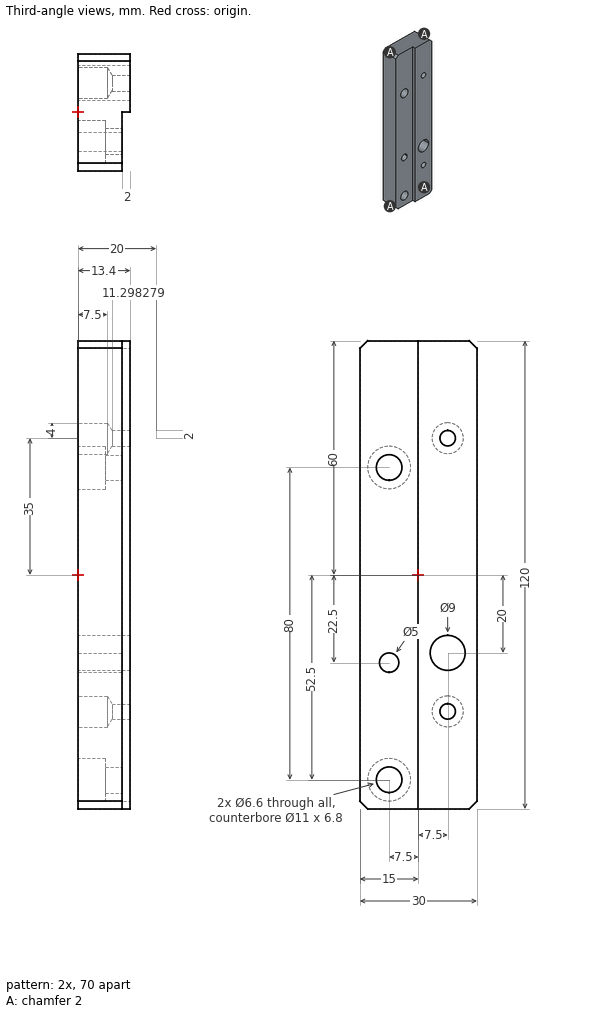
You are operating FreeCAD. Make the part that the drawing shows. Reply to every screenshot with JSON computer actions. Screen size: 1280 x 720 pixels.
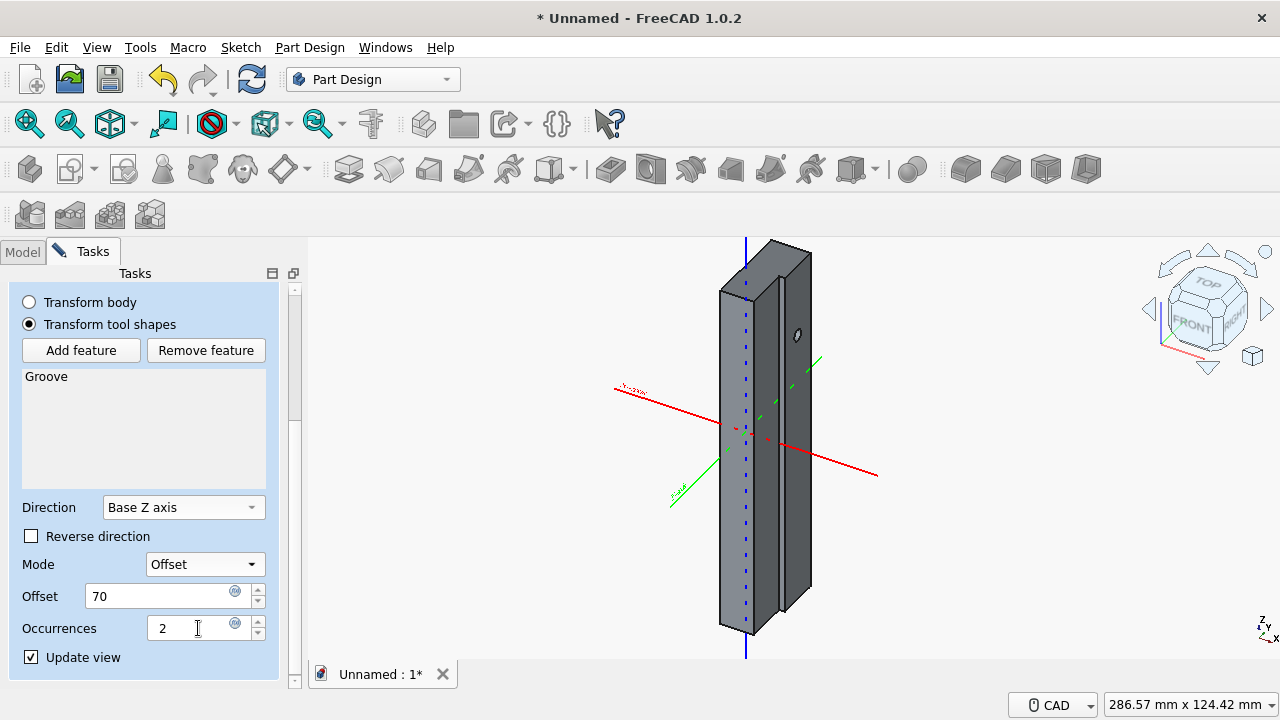
{"action": "left_click", "coordinate": [30, 536]}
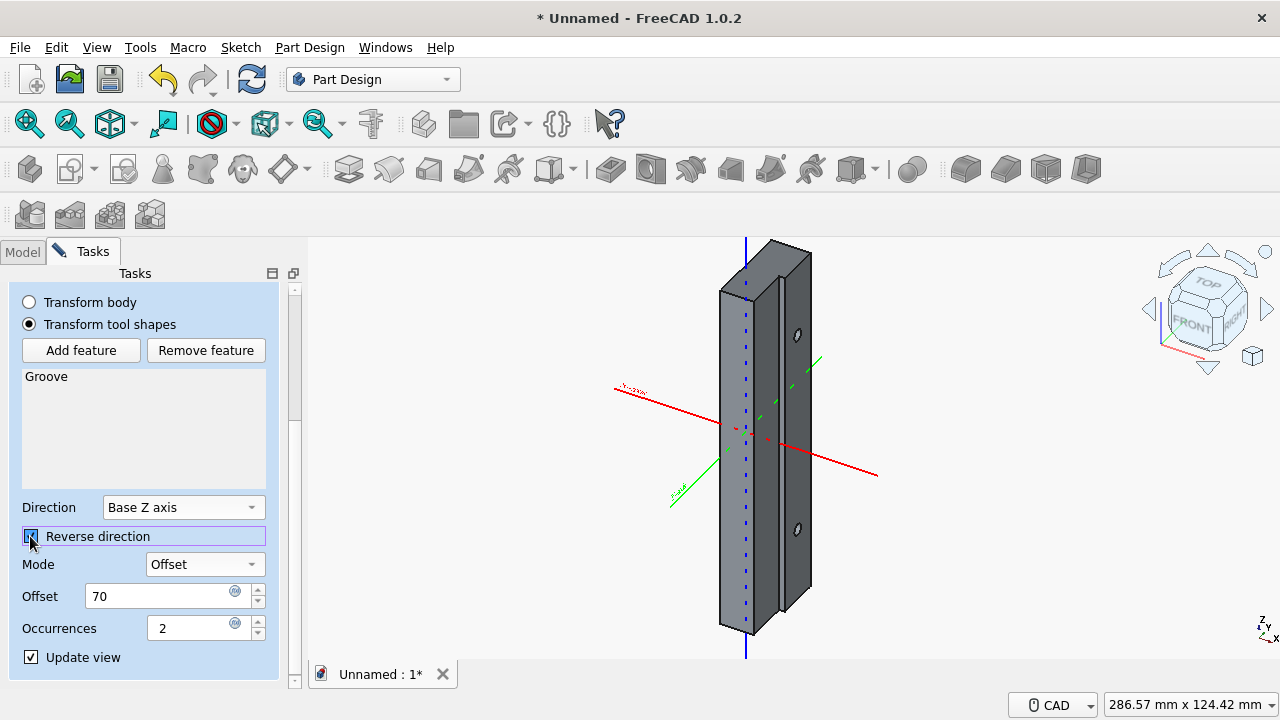
{"action": "scroll", "coordinate": [295, 486], "scroll_direction": "up", "scroll_amount": 5}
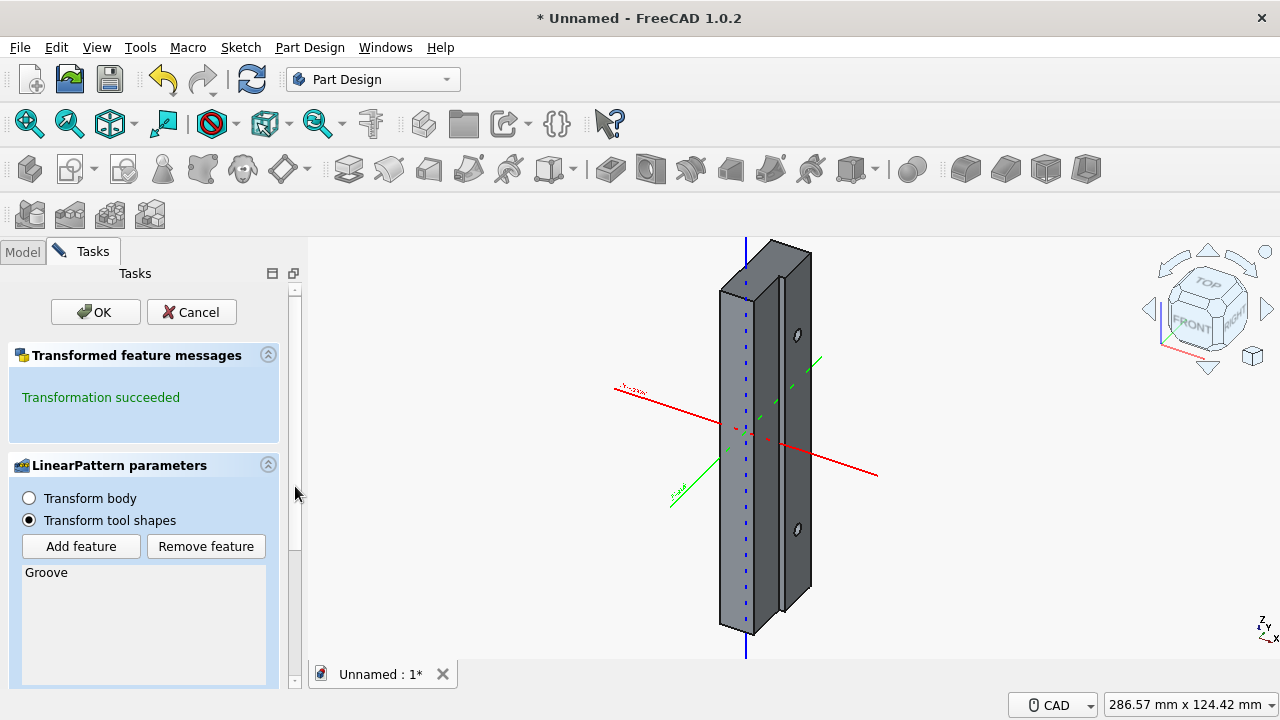
{"action": "left_click", "coordinate": [96, 312]}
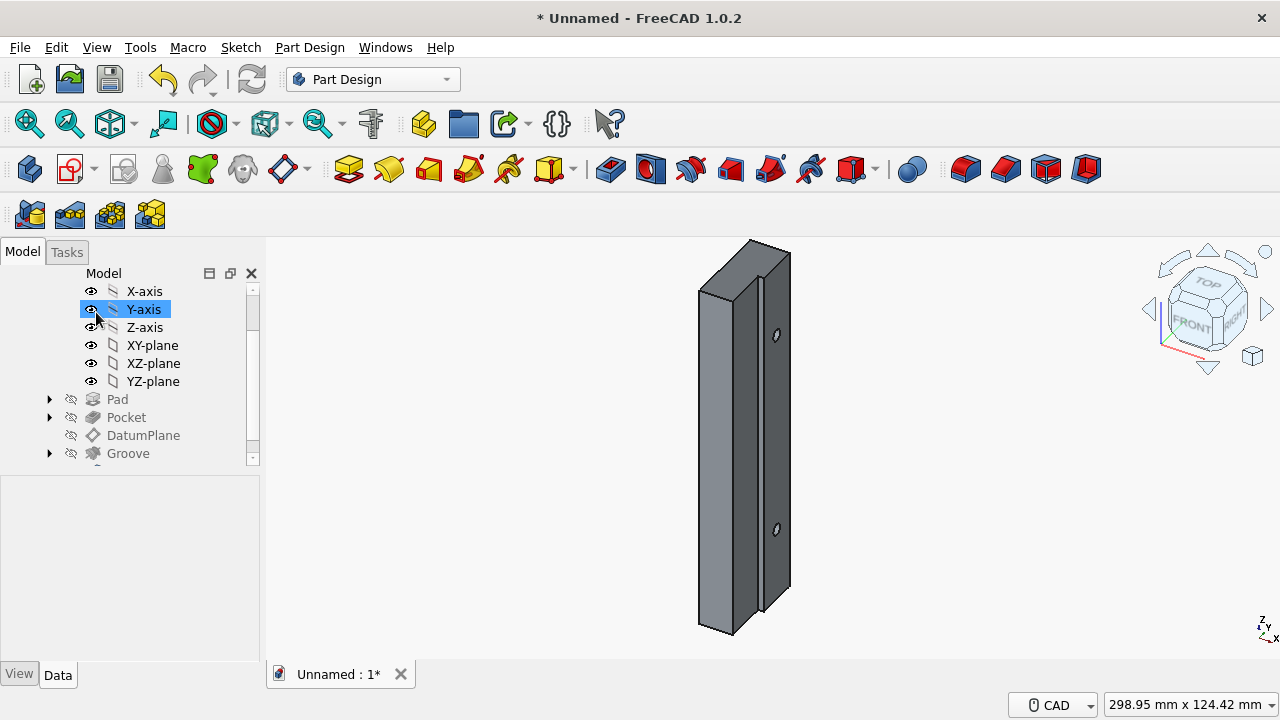
{"action": "left_click", "coordinate": [777, 289]}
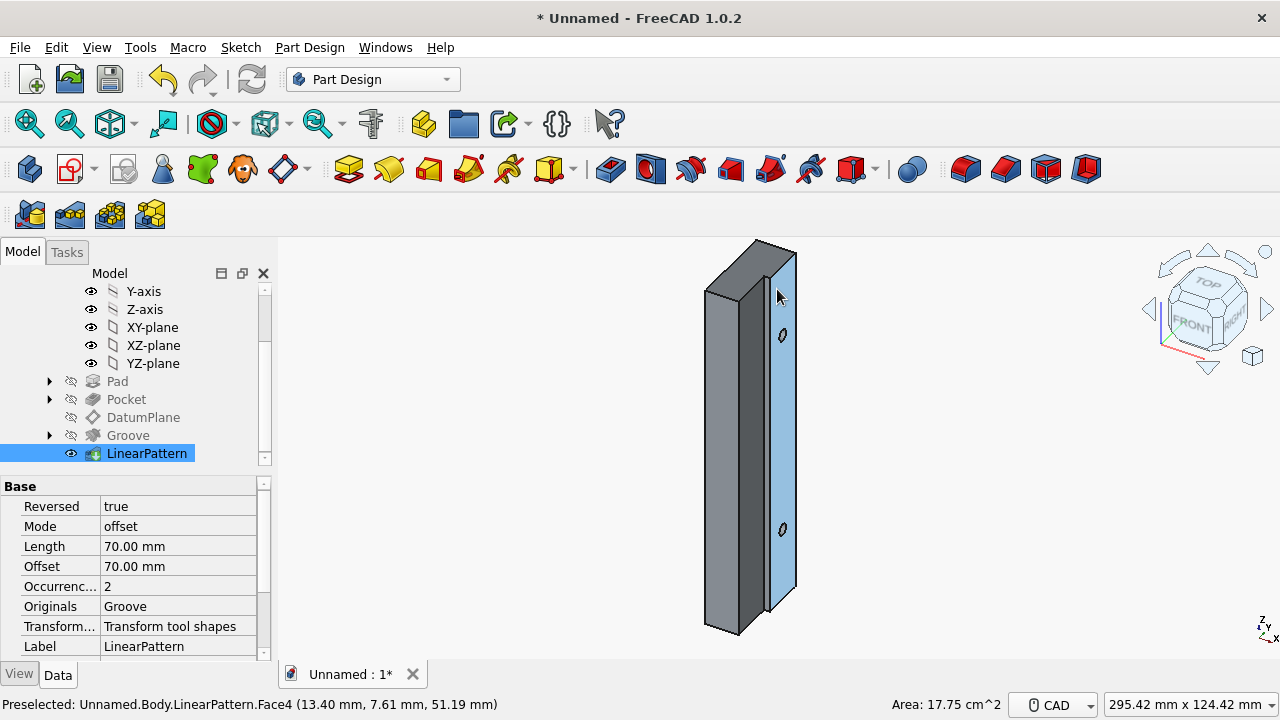
{"action": "left_click", "coordinate": [70, 170]}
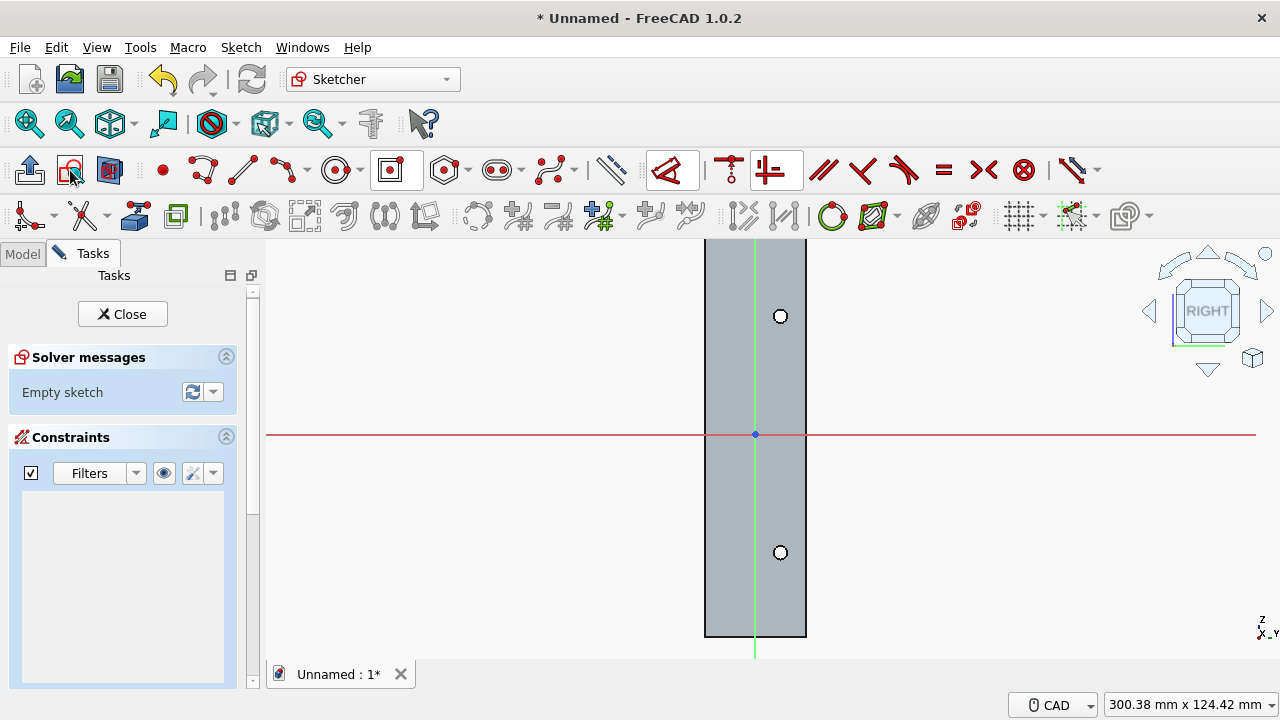
{"action": "scroll", "coordinate": [790, 509], "scroll_direction": "up", "scroll_amount": 11}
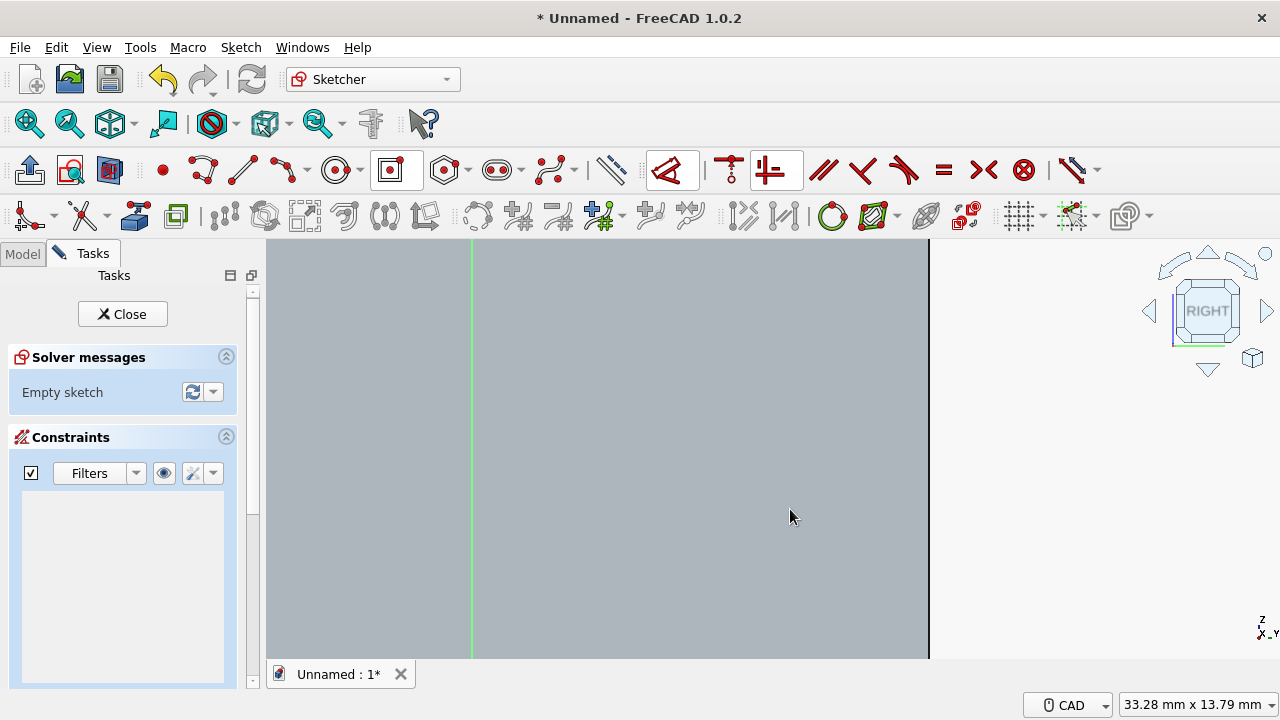
{"action": "left_click", "coordinate": [336, 170]}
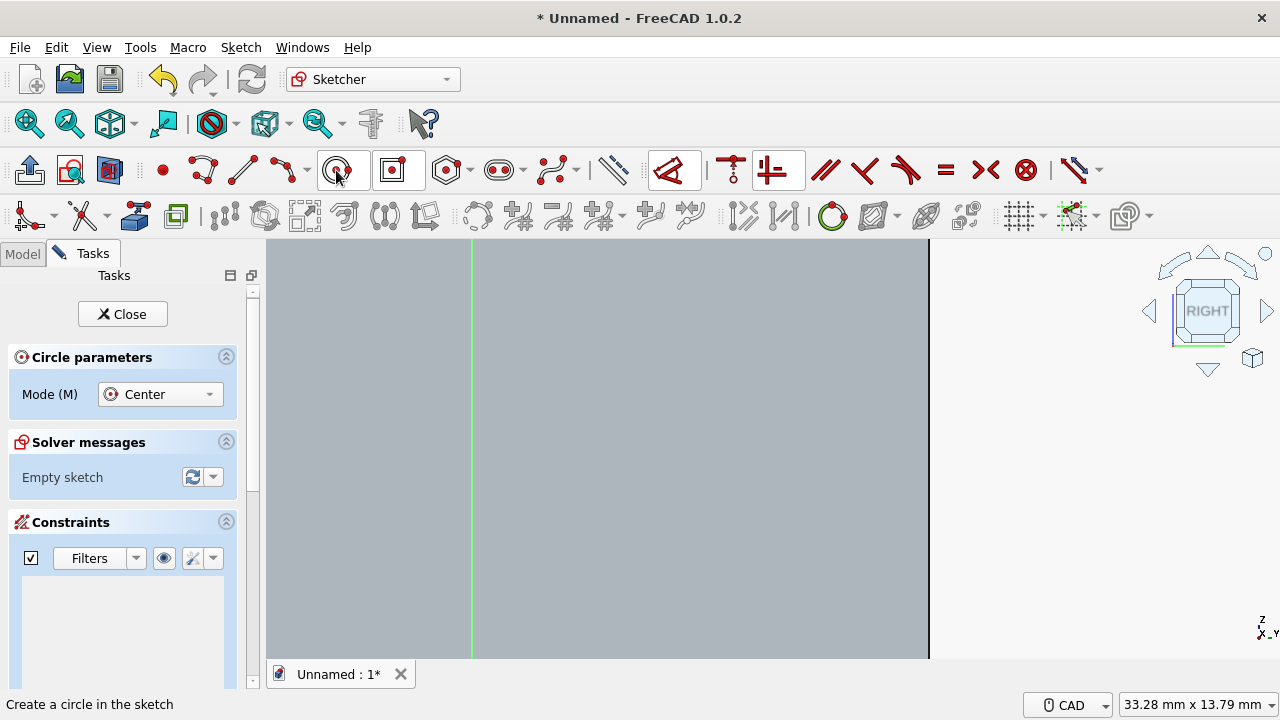
{"action": "left_click", "coordinate": [700, 442]}
{"action": "left_click", "coordinate": [797, 345]}
{"action": "key", "text": "Escape"}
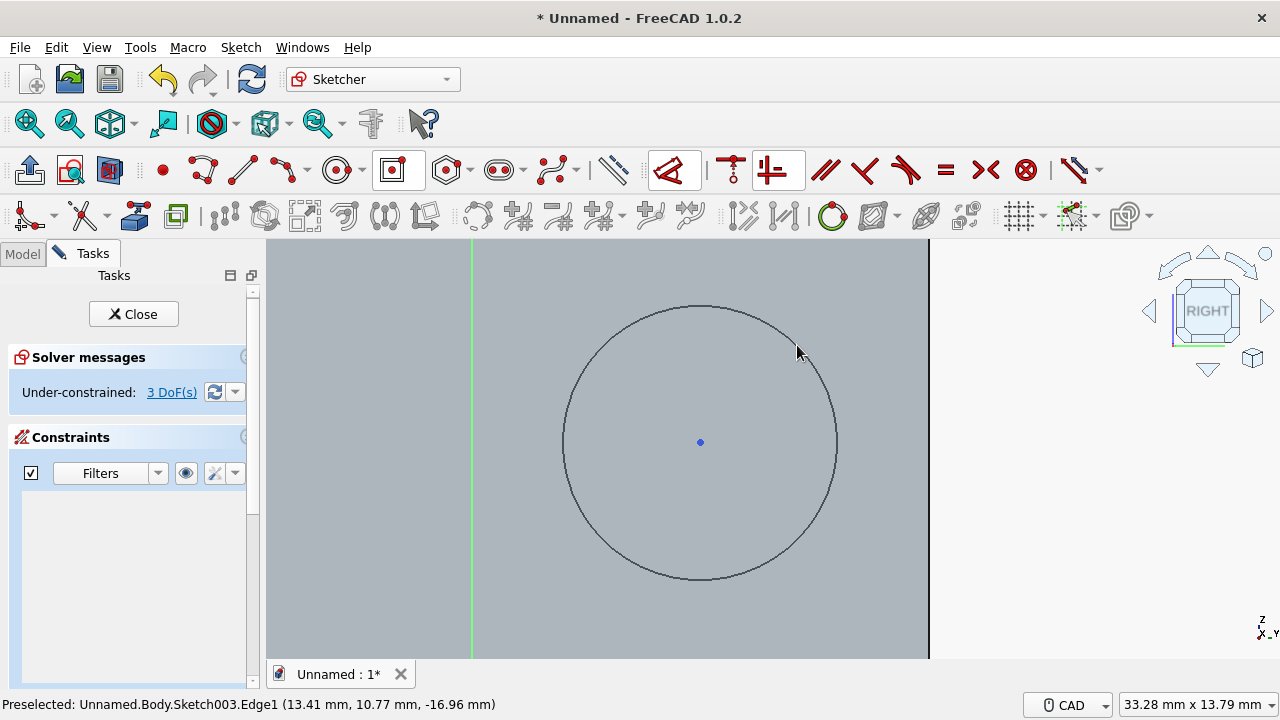
{"action": "left_click", "coordinate": [797, 346]}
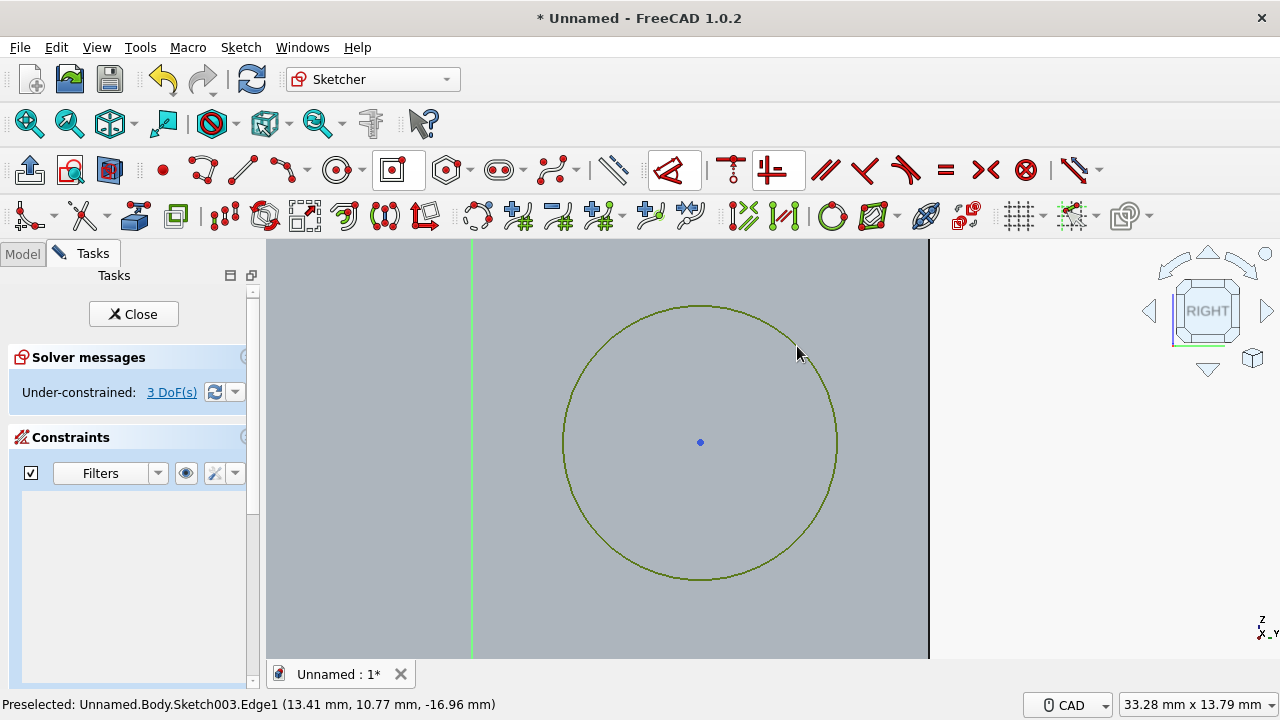
{"action": "key", "text": "k o"}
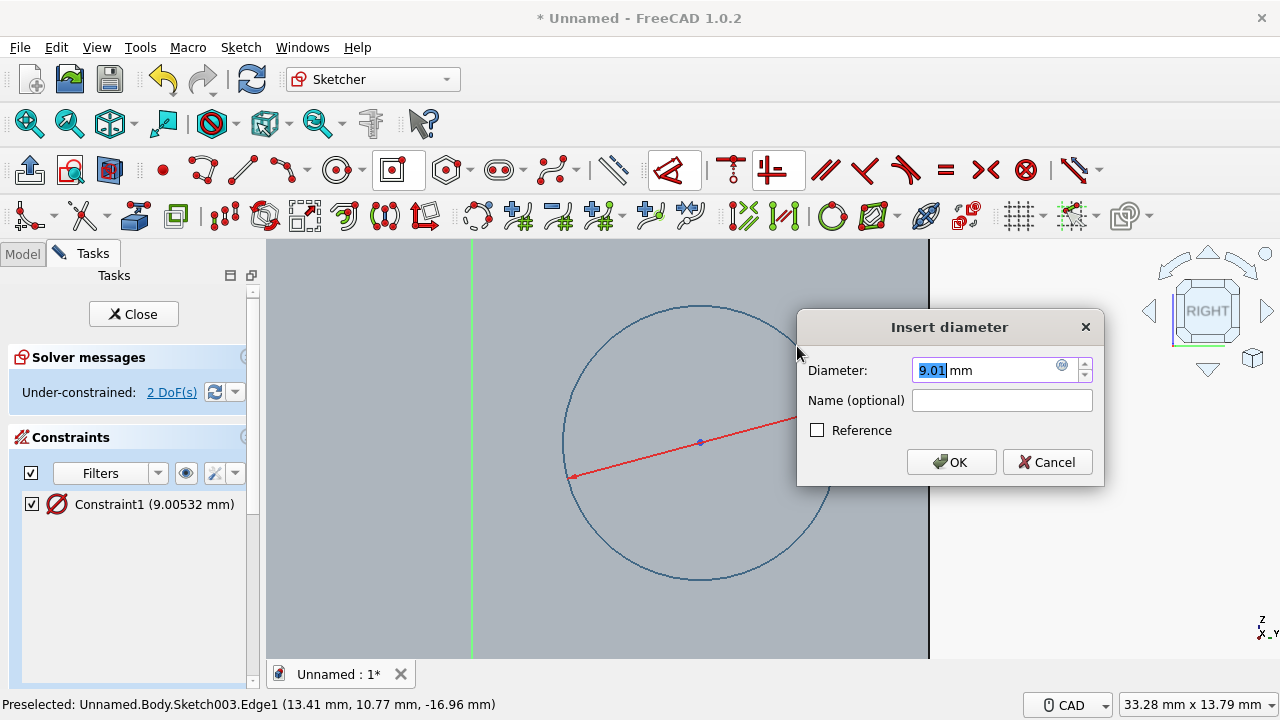
{"action": "type", "text": "9"}
{"action": "key", "text": "Return"}